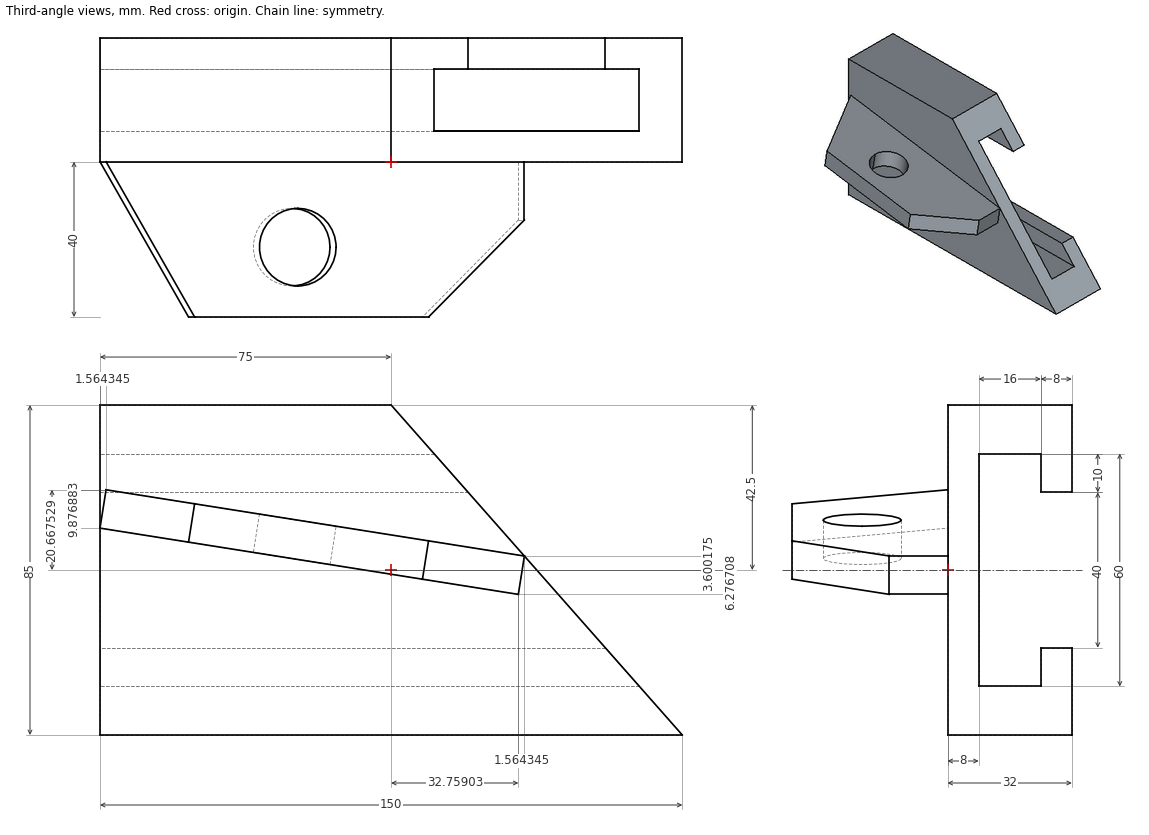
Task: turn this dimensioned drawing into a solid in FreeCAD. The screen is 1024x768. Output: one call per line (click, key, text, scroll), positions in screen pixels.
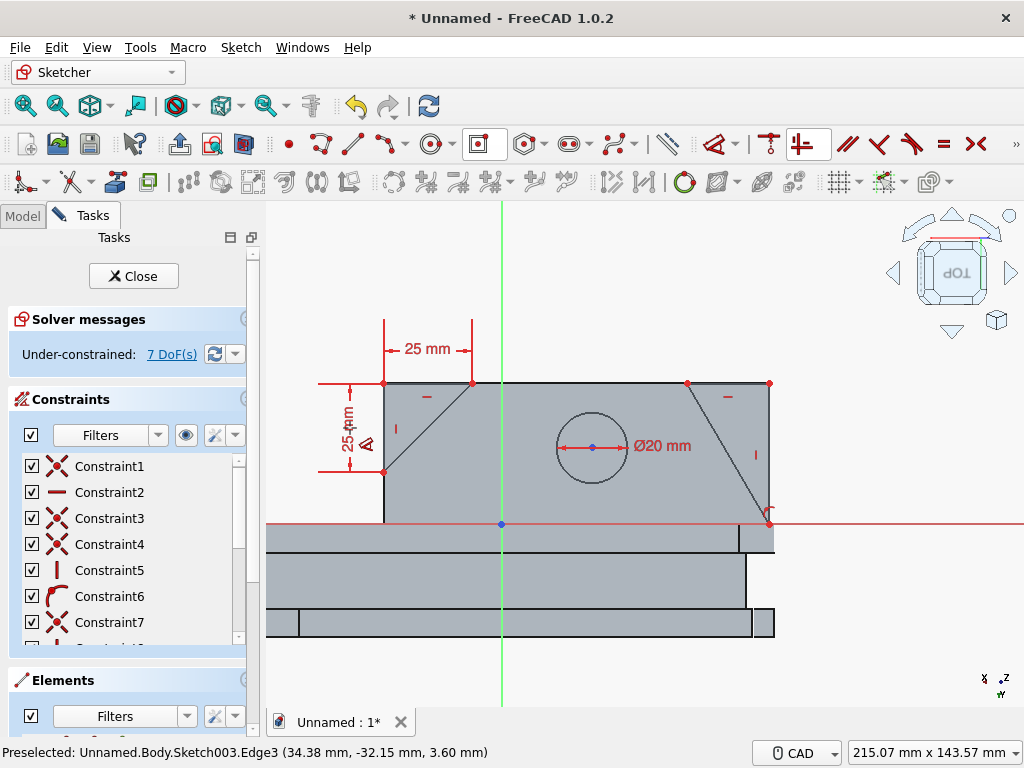
click(769, 482)
click(803, 454)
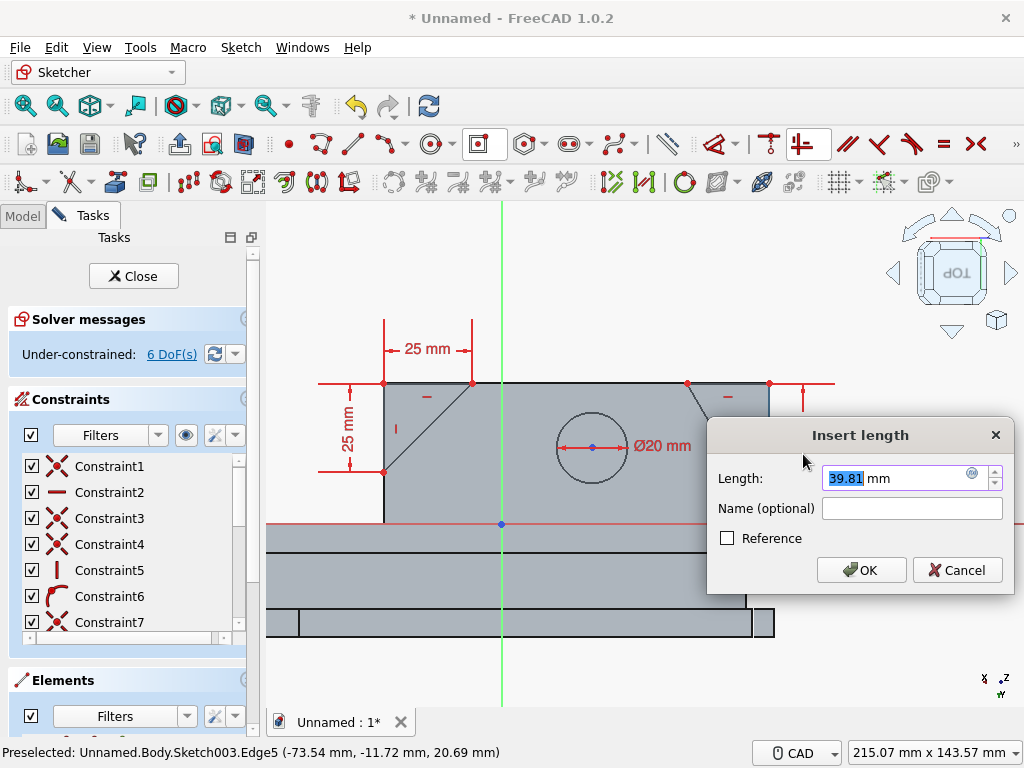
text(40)
key(Return)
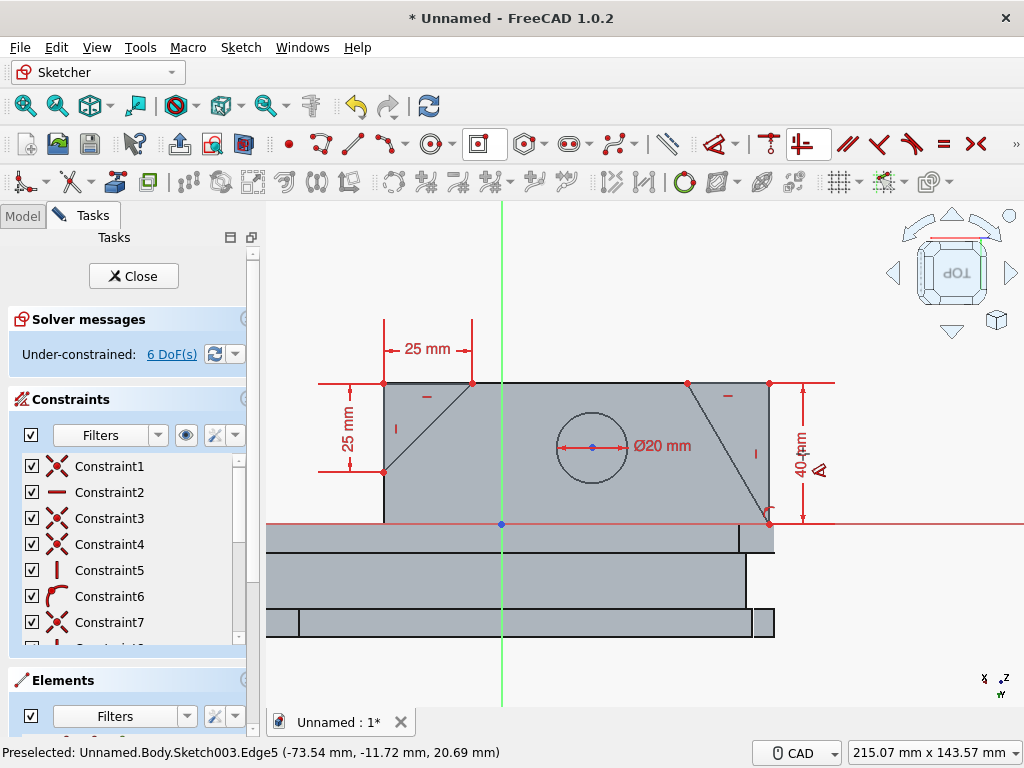
click(592, 448)
click(468, 486)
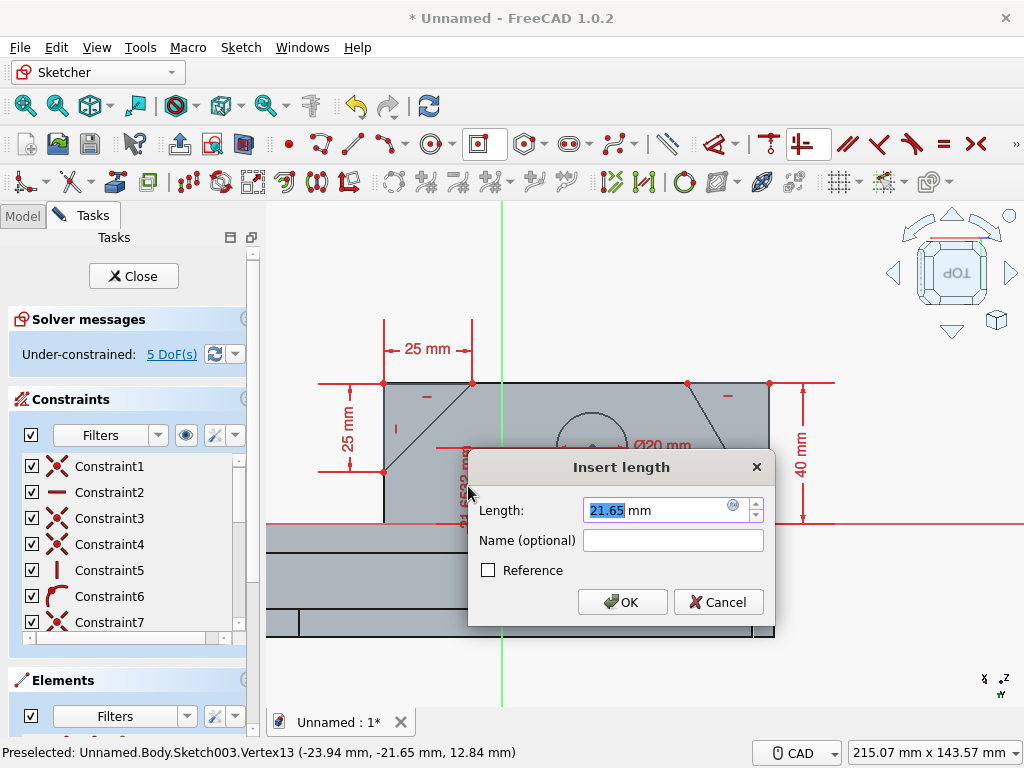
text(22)
key(Return)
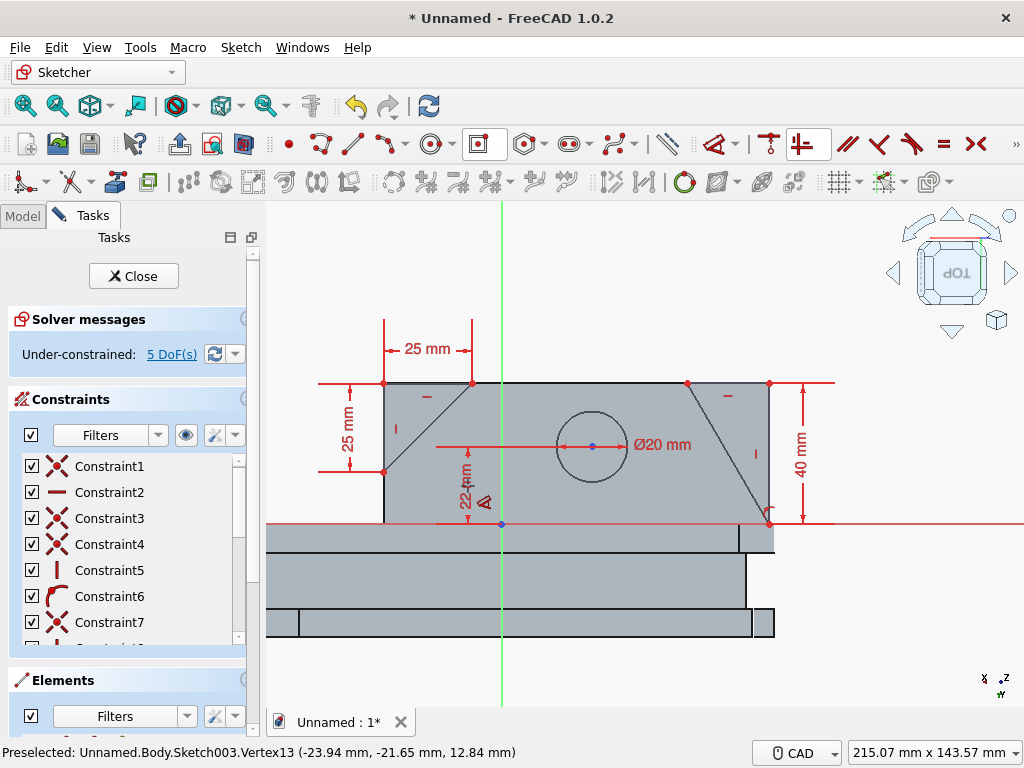
click(384, 472)
click(350, 498)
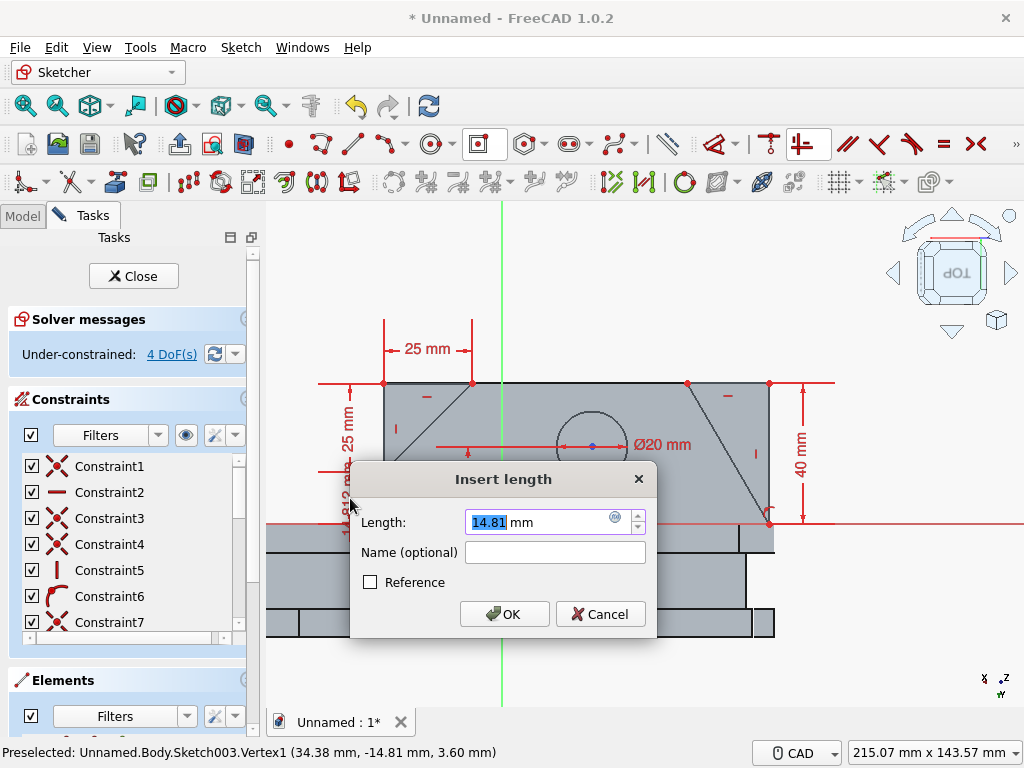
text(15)
key(Return)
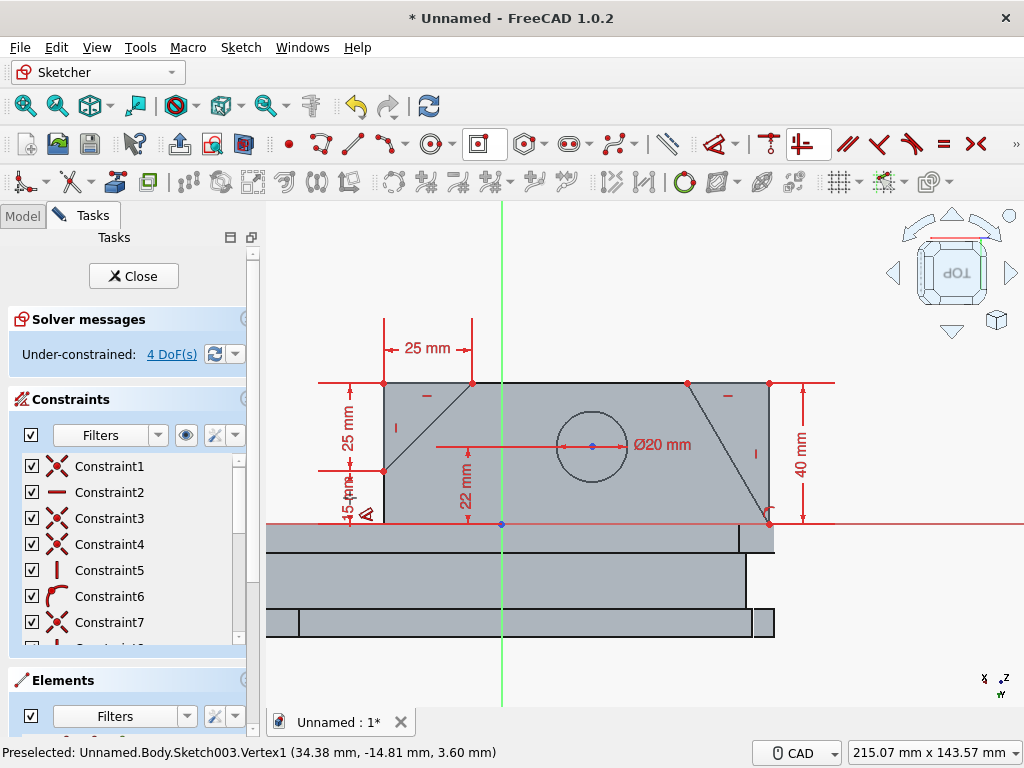
click(769, 383)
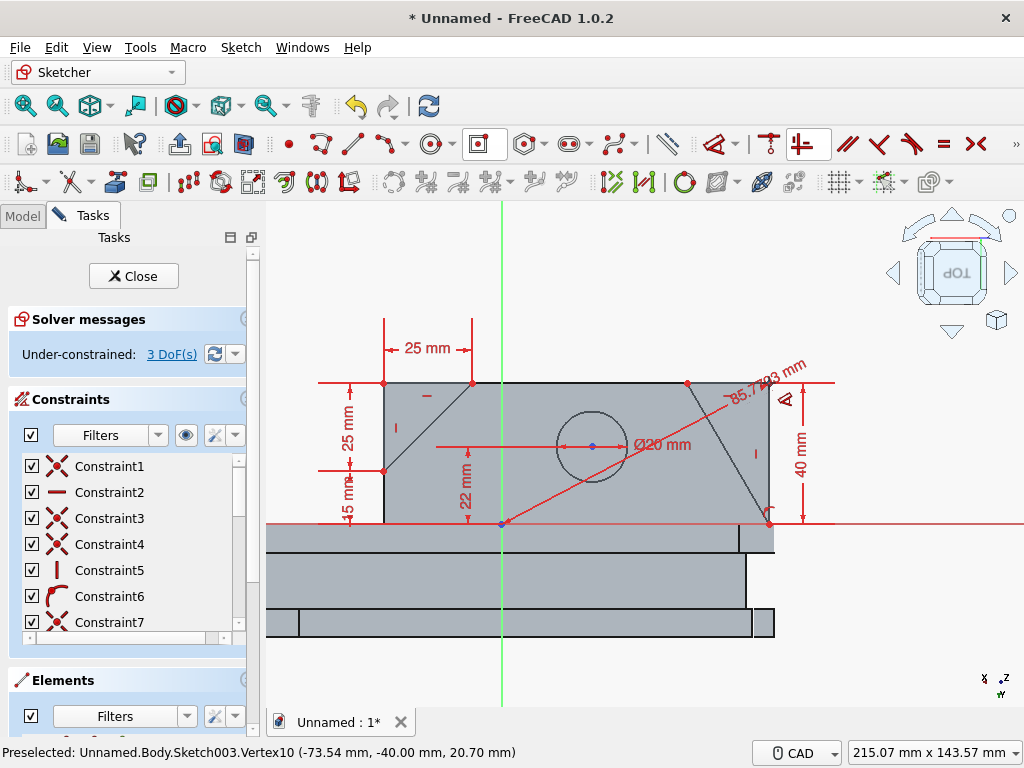
click(592, 447)
click(681, 349)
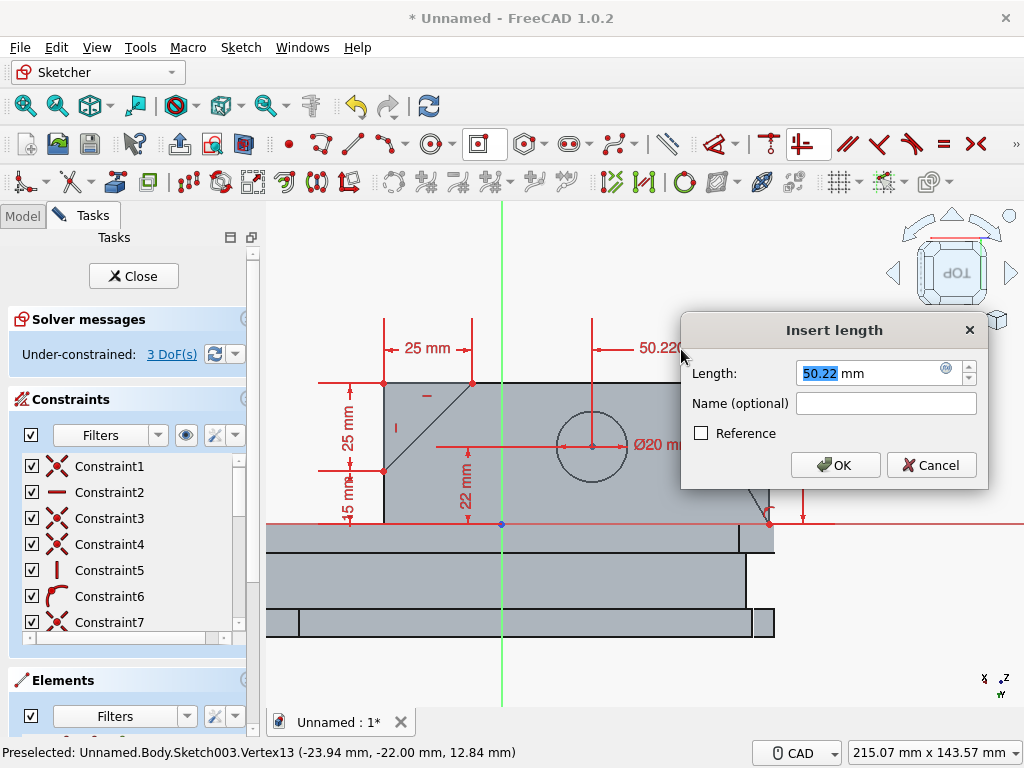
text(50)
key(Return)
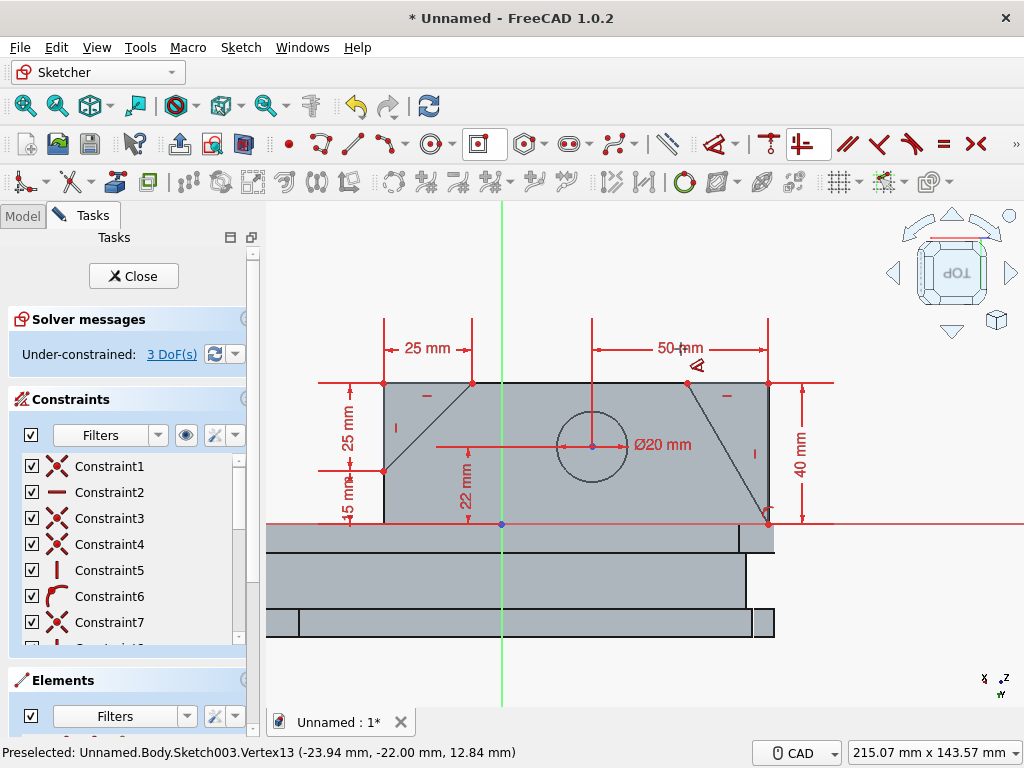
click(744, 383)
click(756, 349)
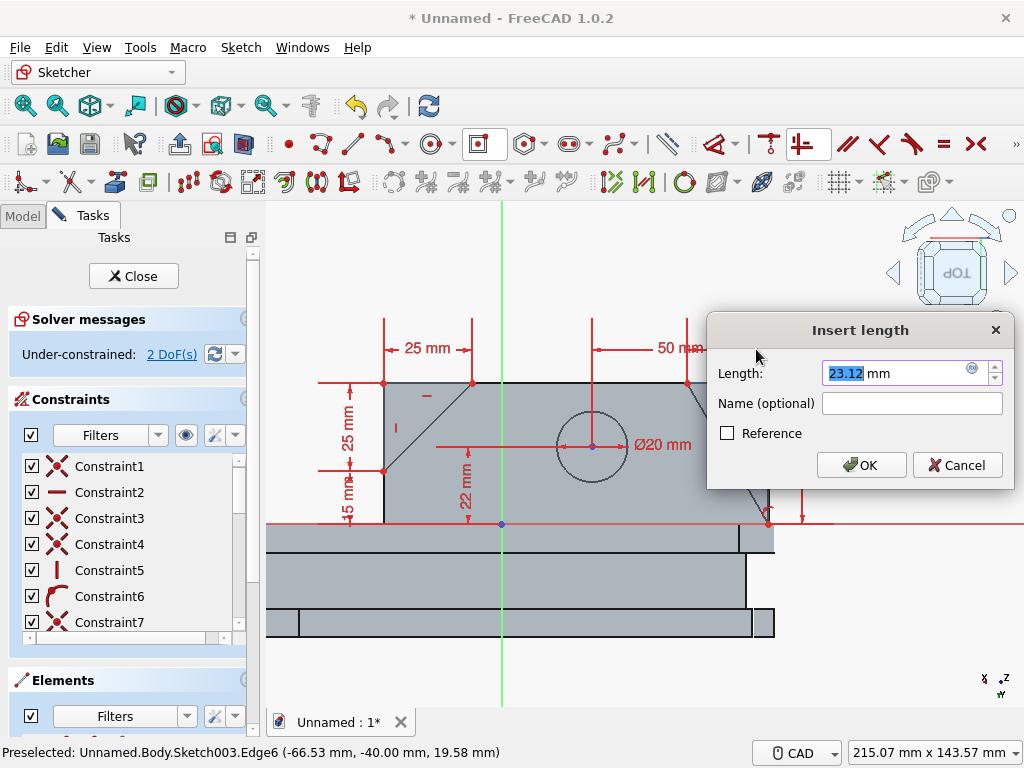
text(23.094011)
key(Return)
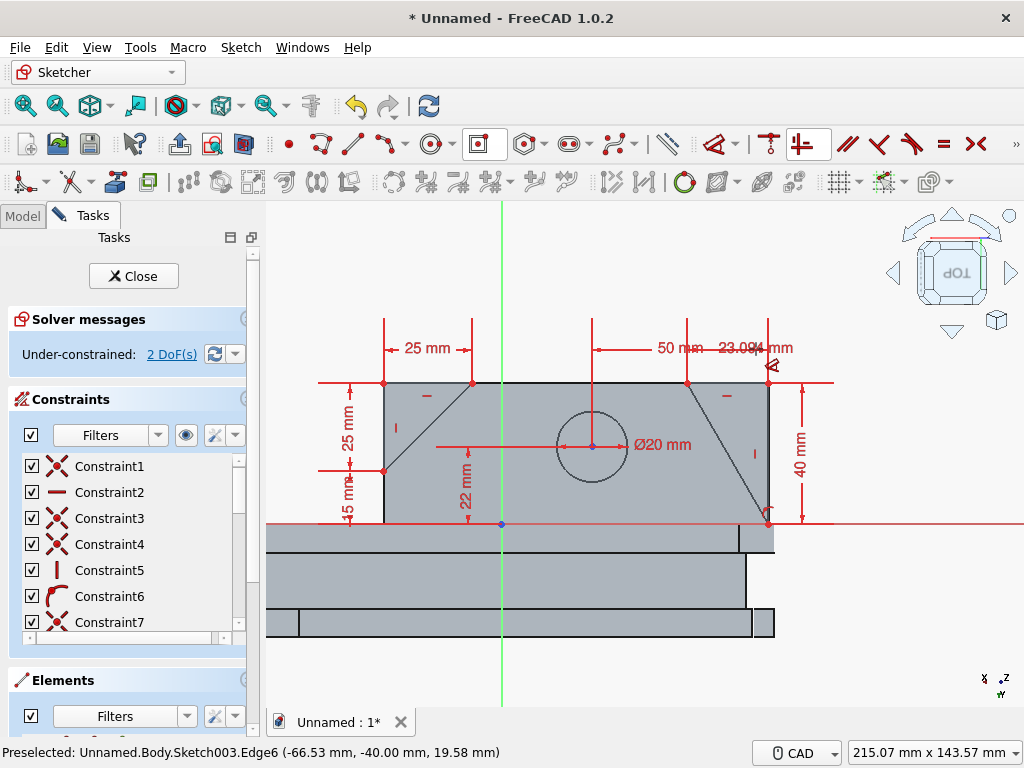
scroll(472, 383, up, 2)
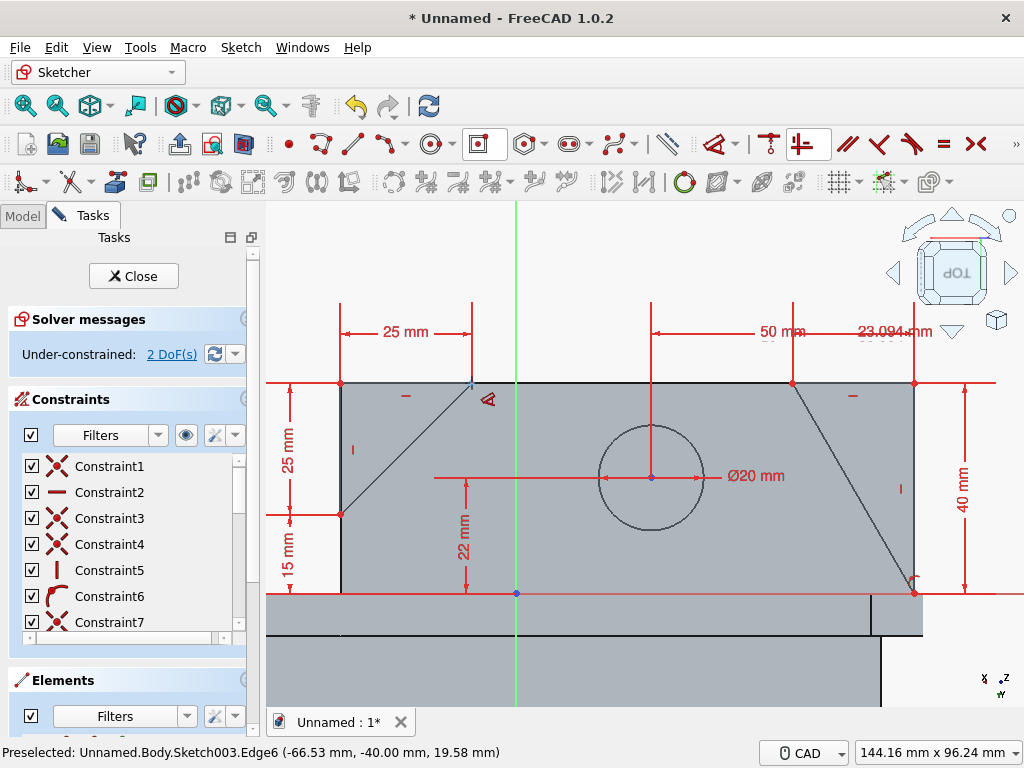
click(472, 383)
click(494, 628)